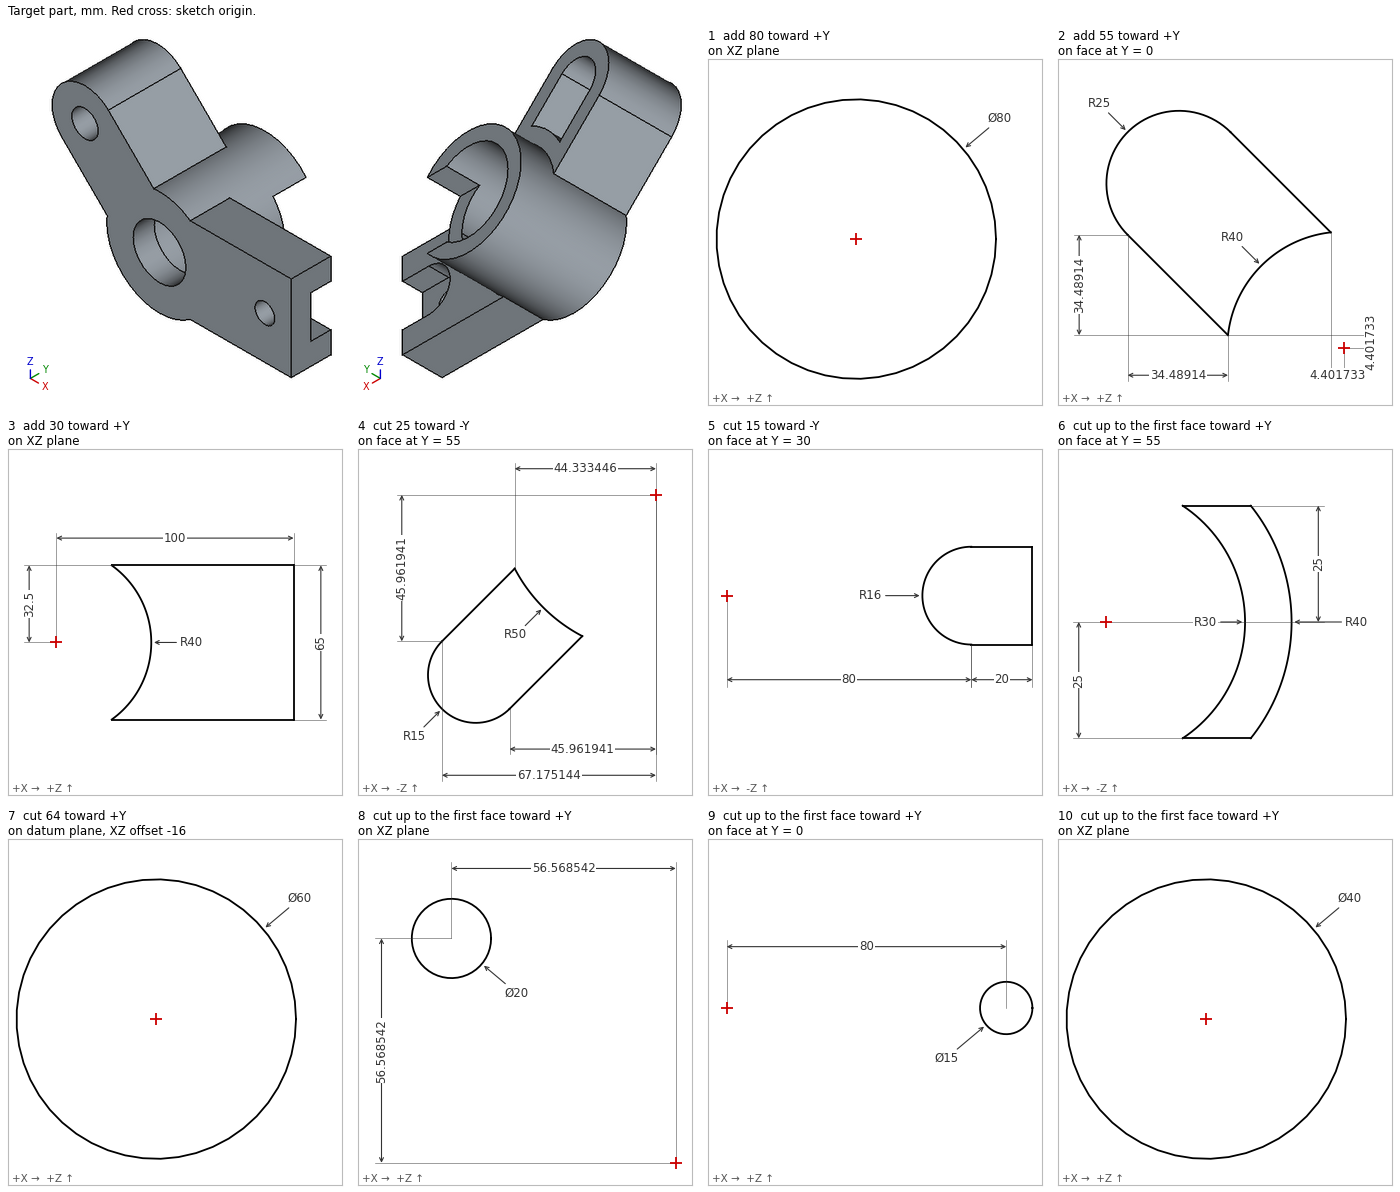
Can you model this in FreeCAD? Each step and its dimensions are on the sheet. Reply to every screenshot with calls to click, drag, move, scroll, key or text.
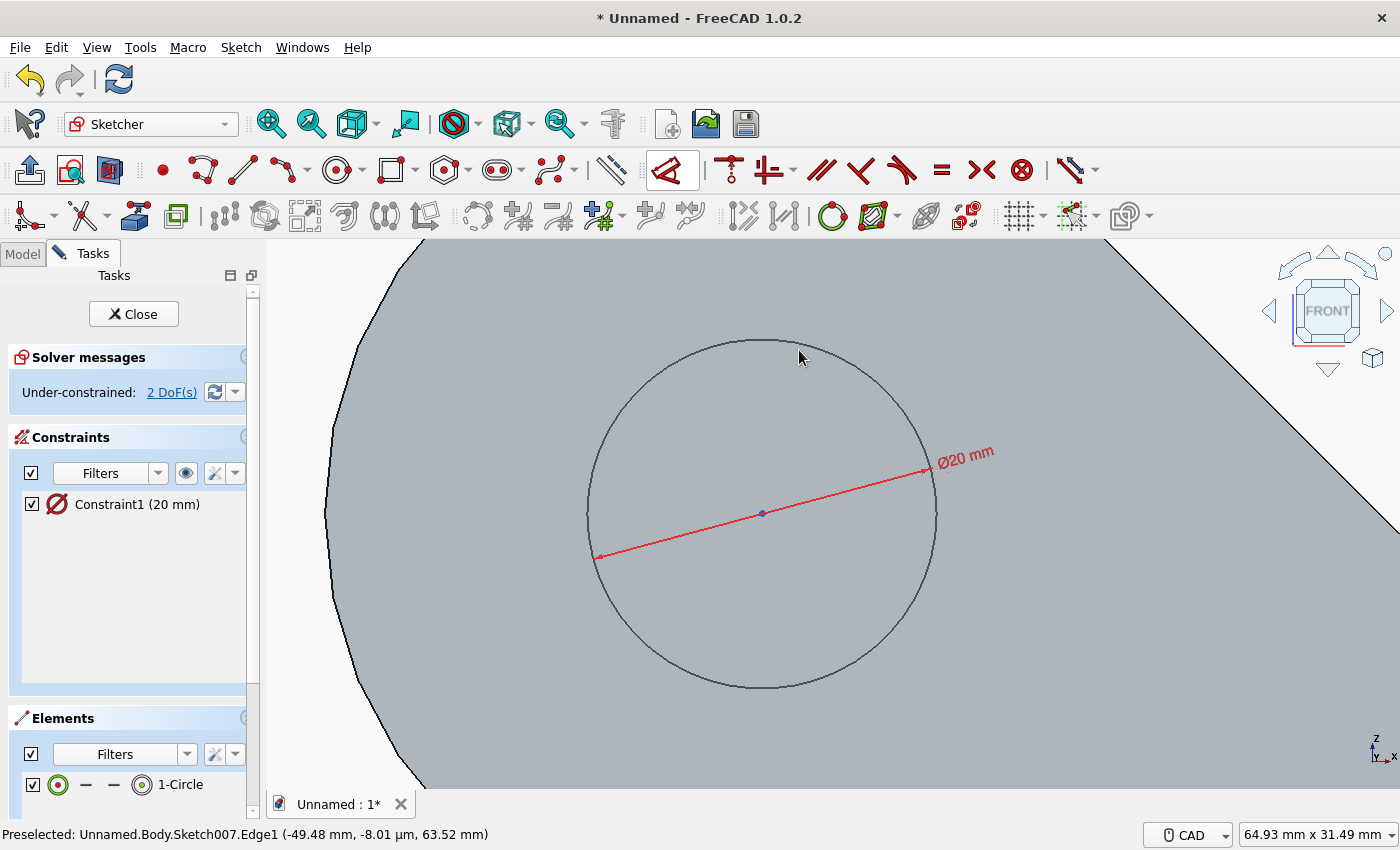
click(762, 514)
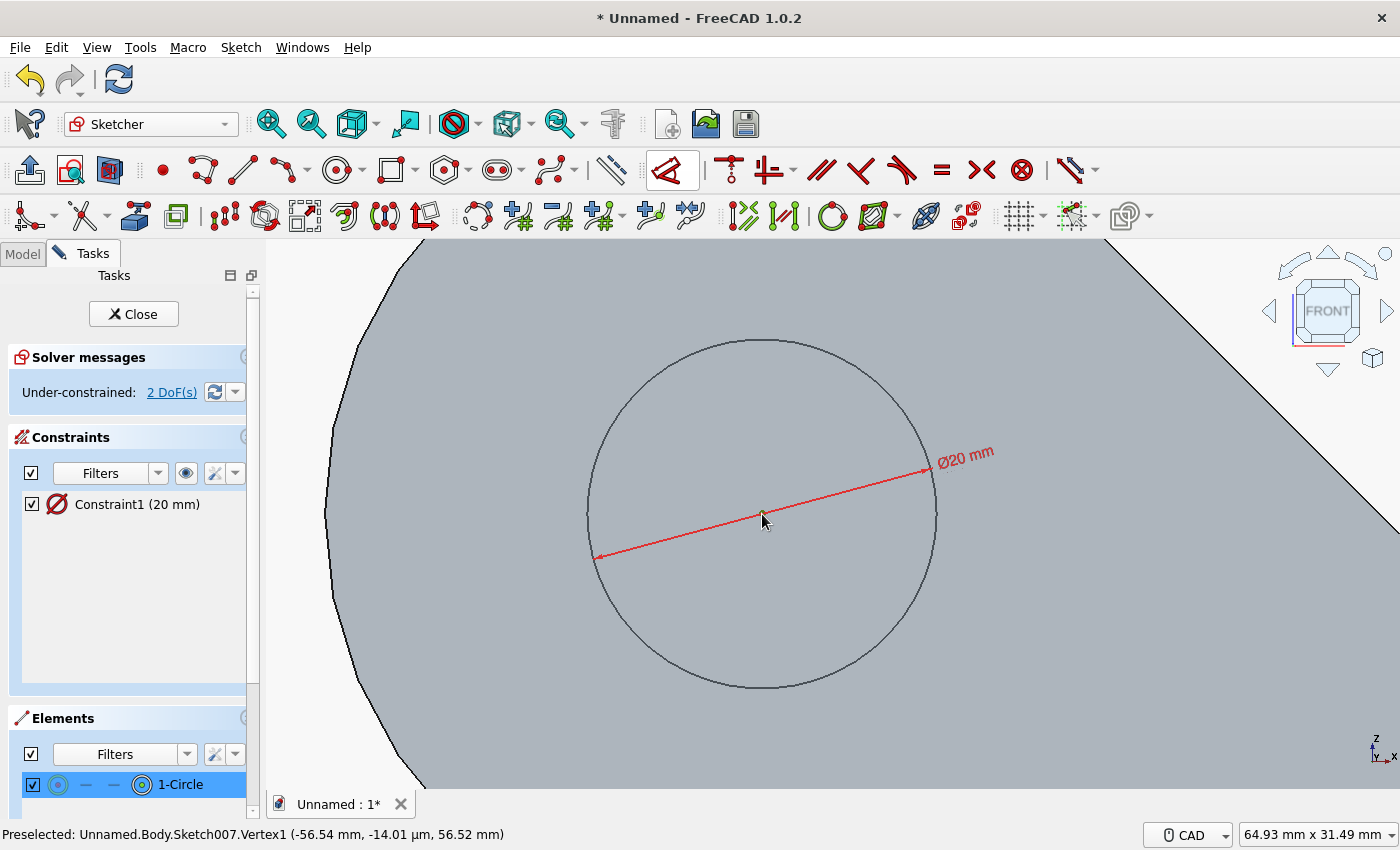
click(694, 170)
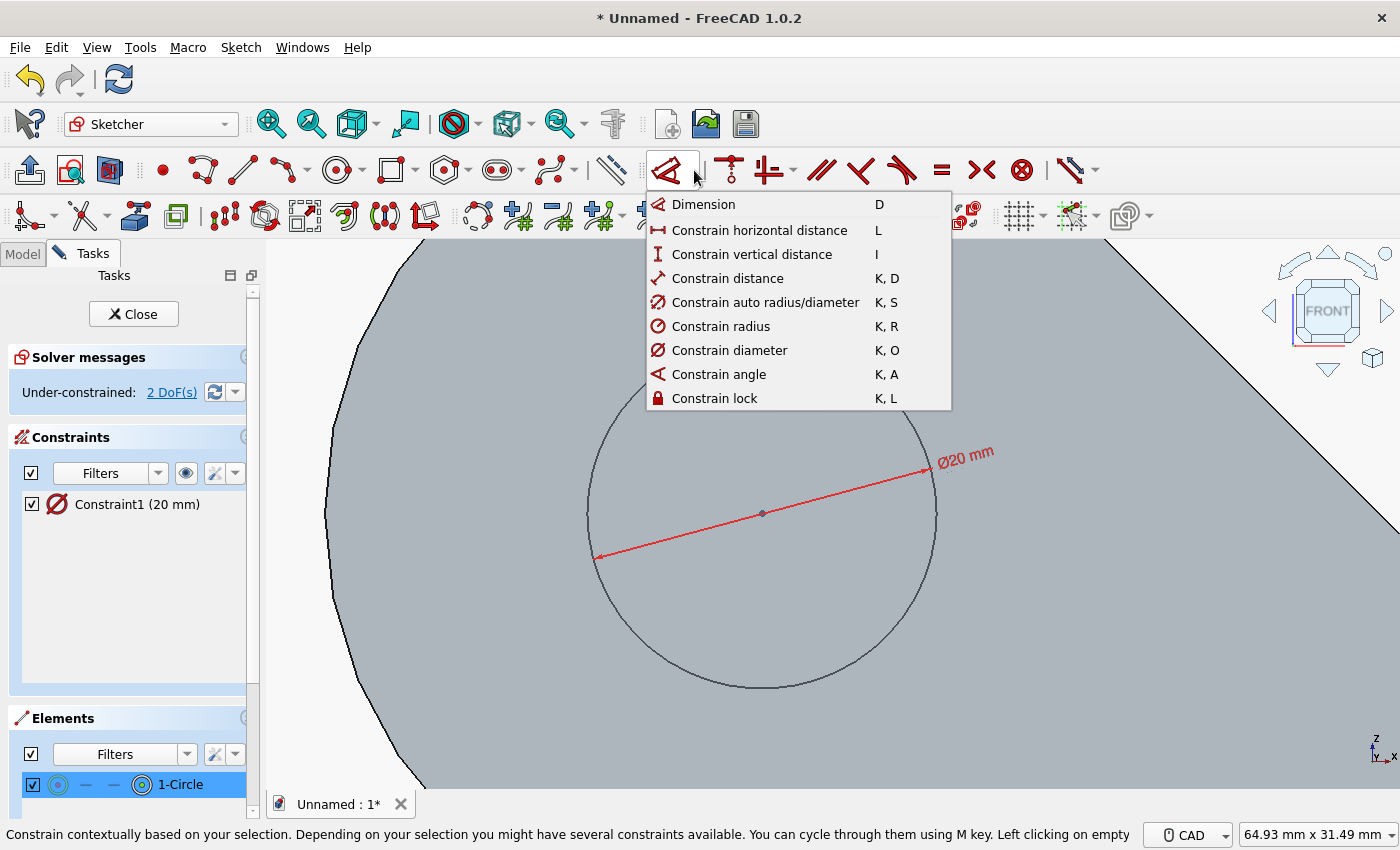
click(799, 230)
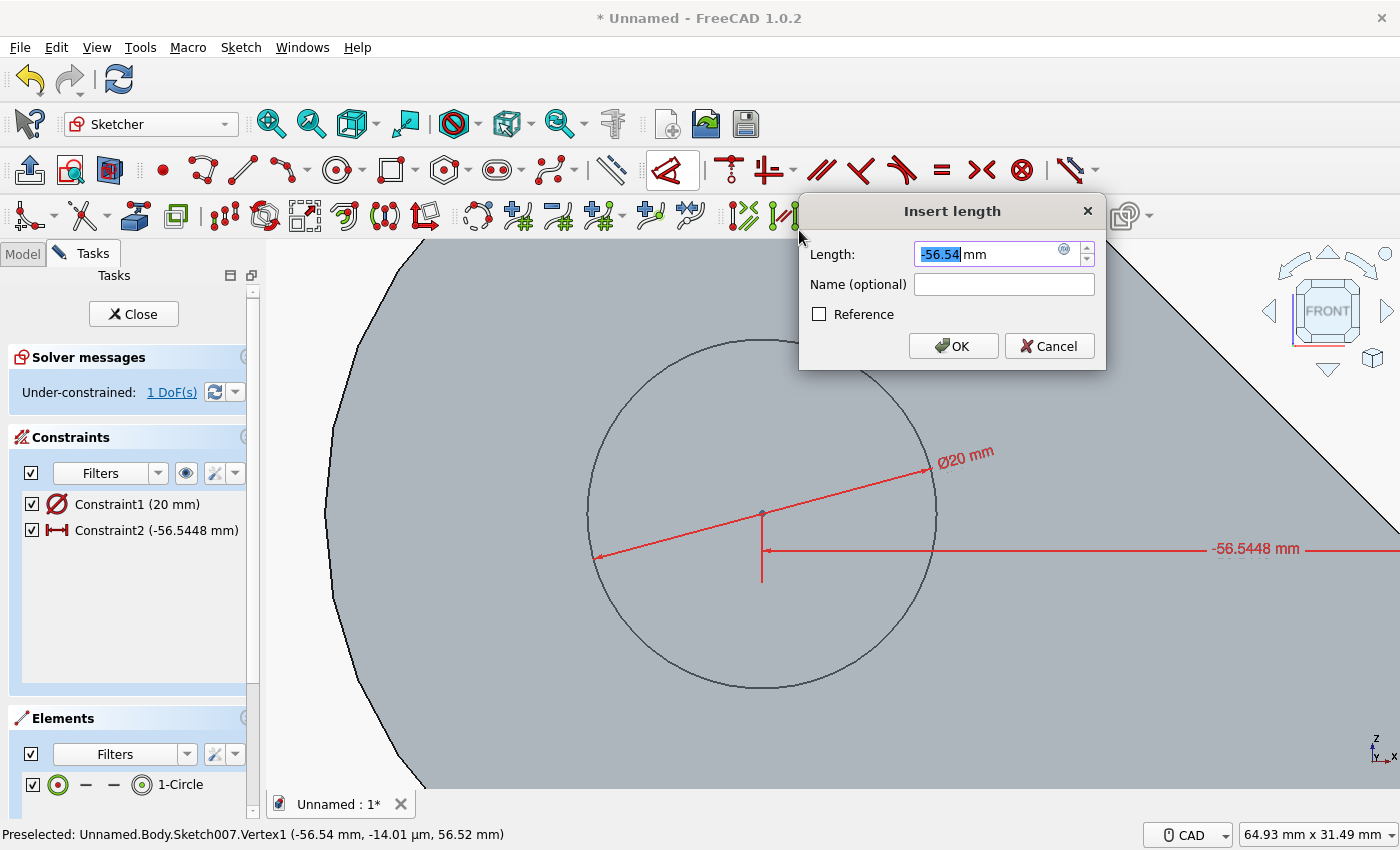
text(-56.568542)
key(Return)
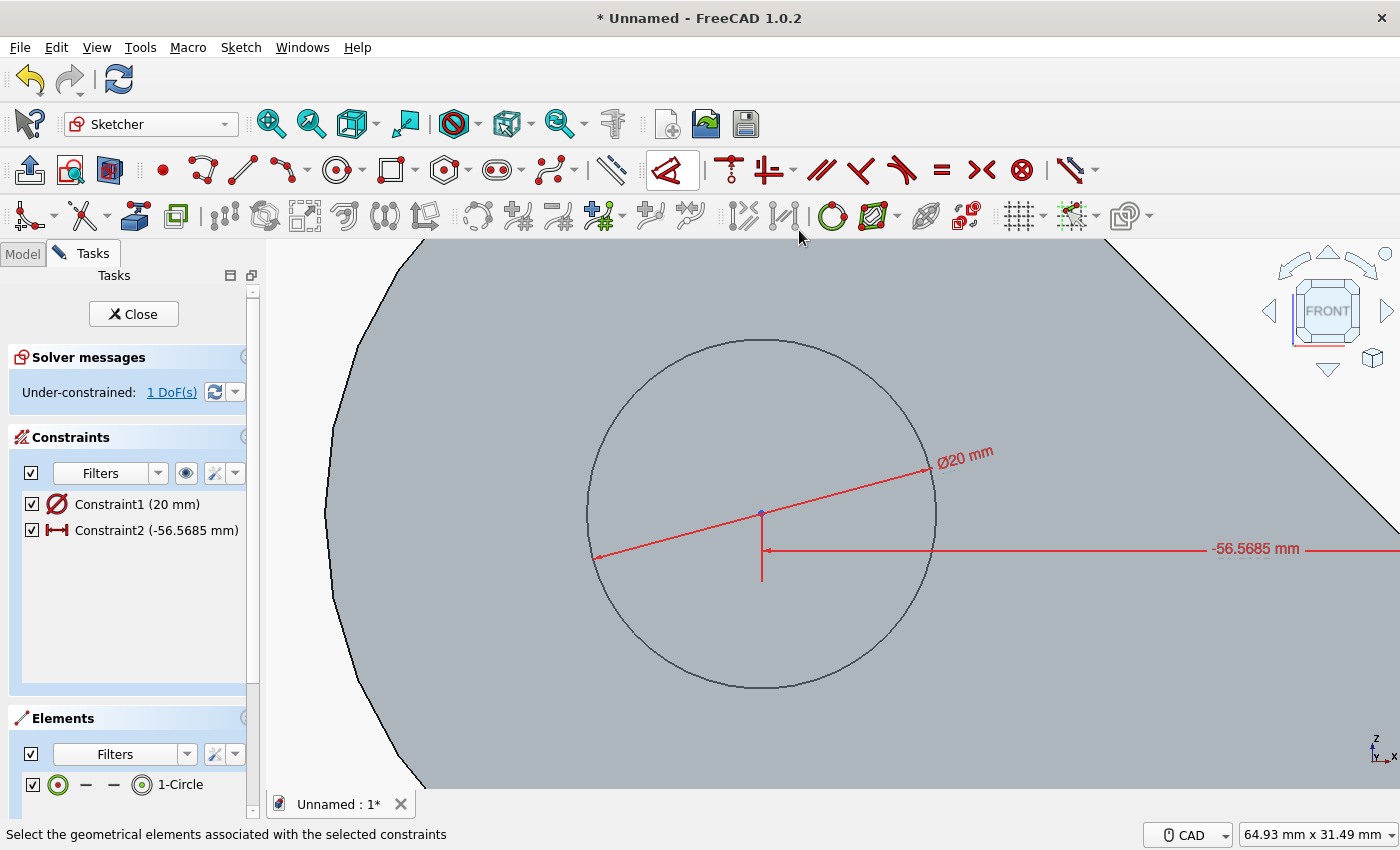
click(762, 514)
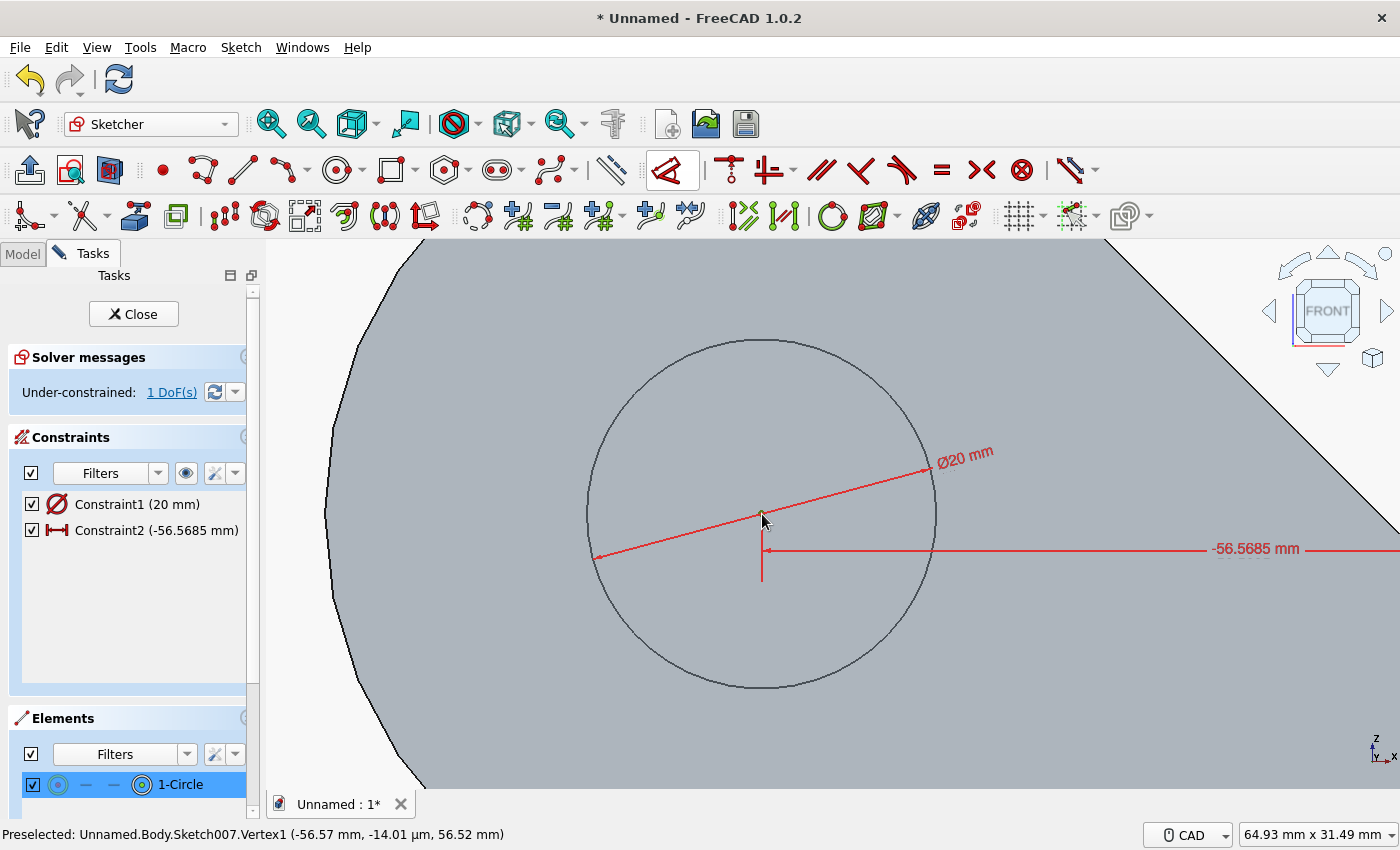
key(i)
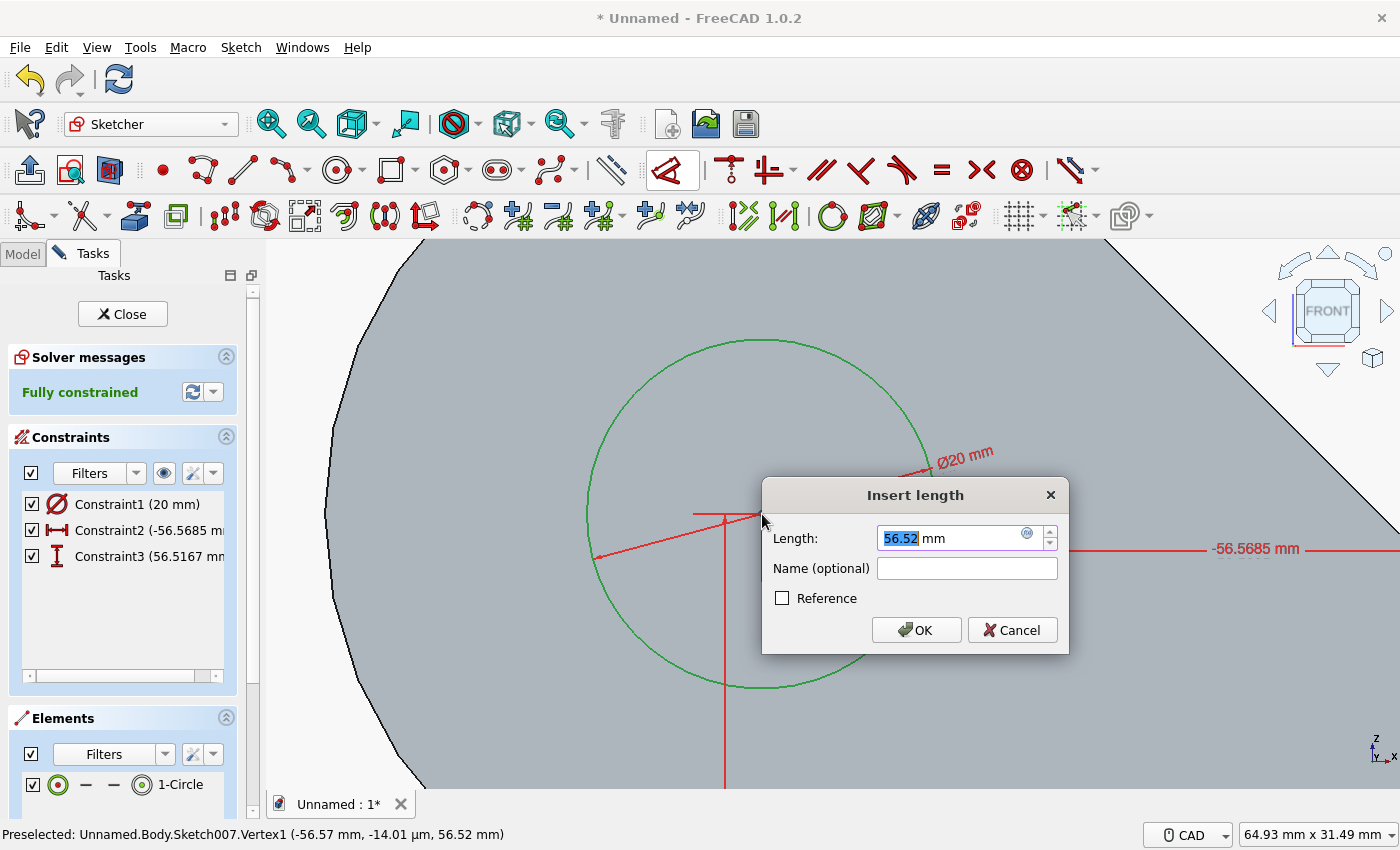
text(56.568542)
key(Return)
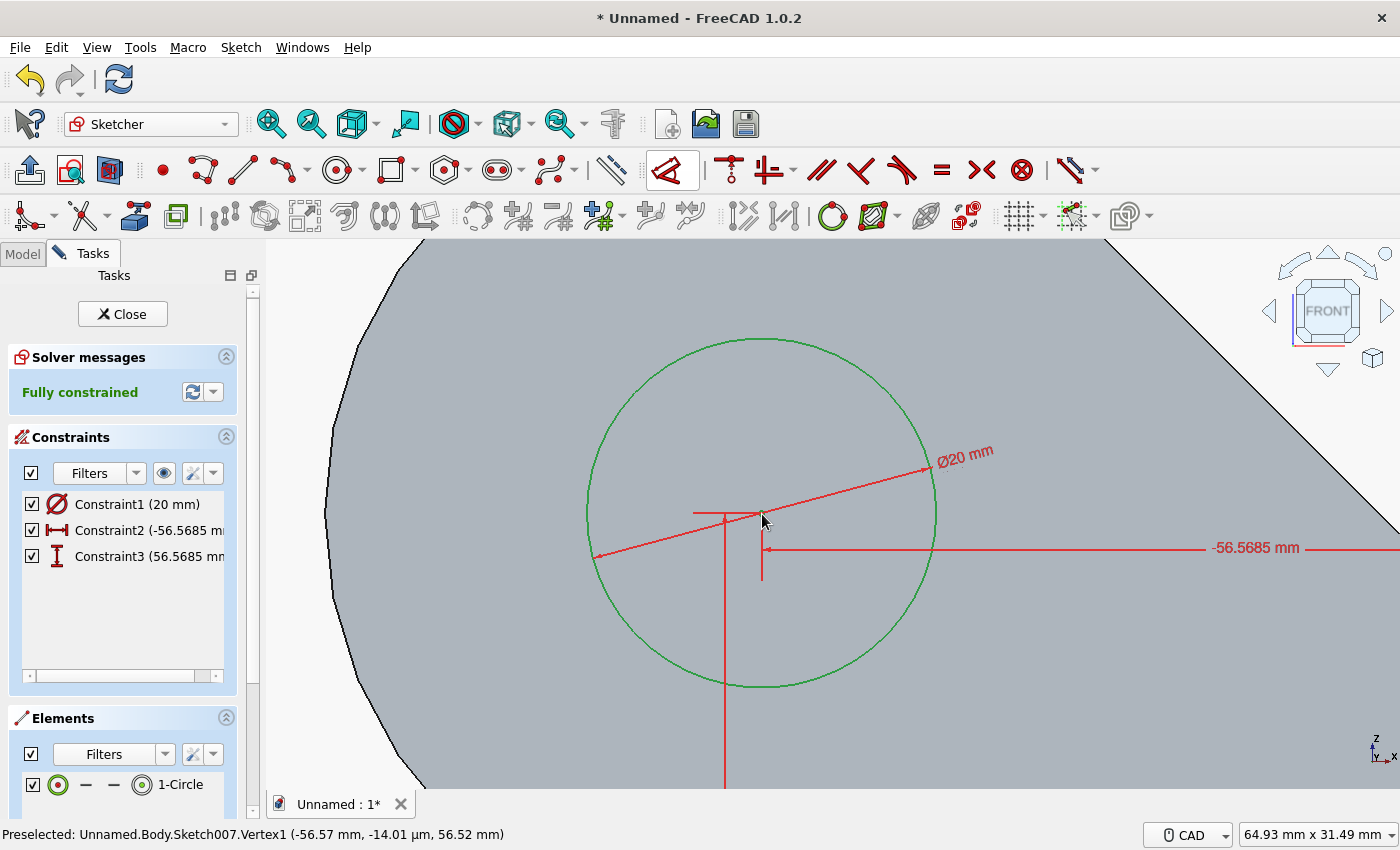
click(123, 314)